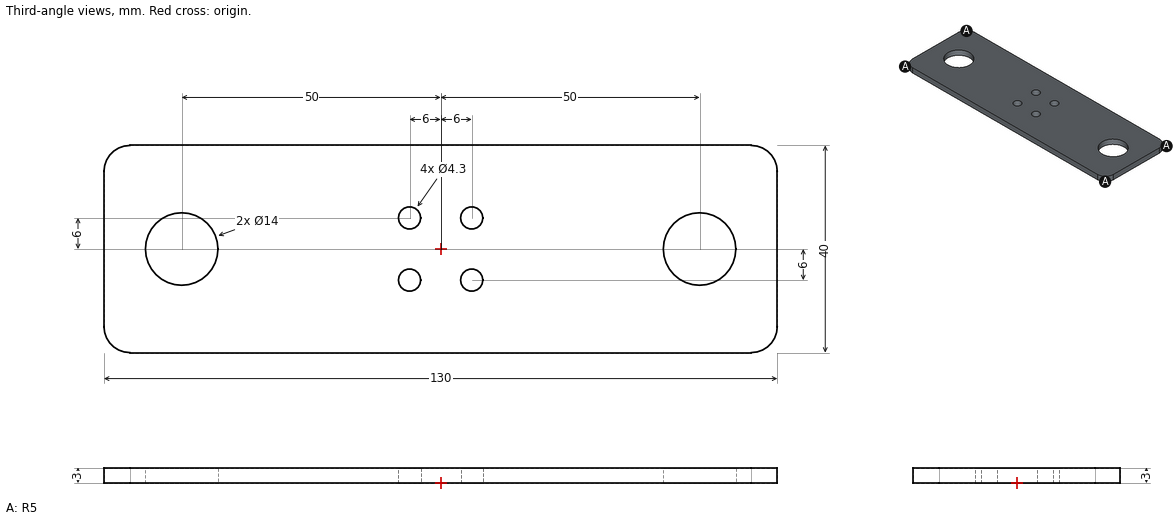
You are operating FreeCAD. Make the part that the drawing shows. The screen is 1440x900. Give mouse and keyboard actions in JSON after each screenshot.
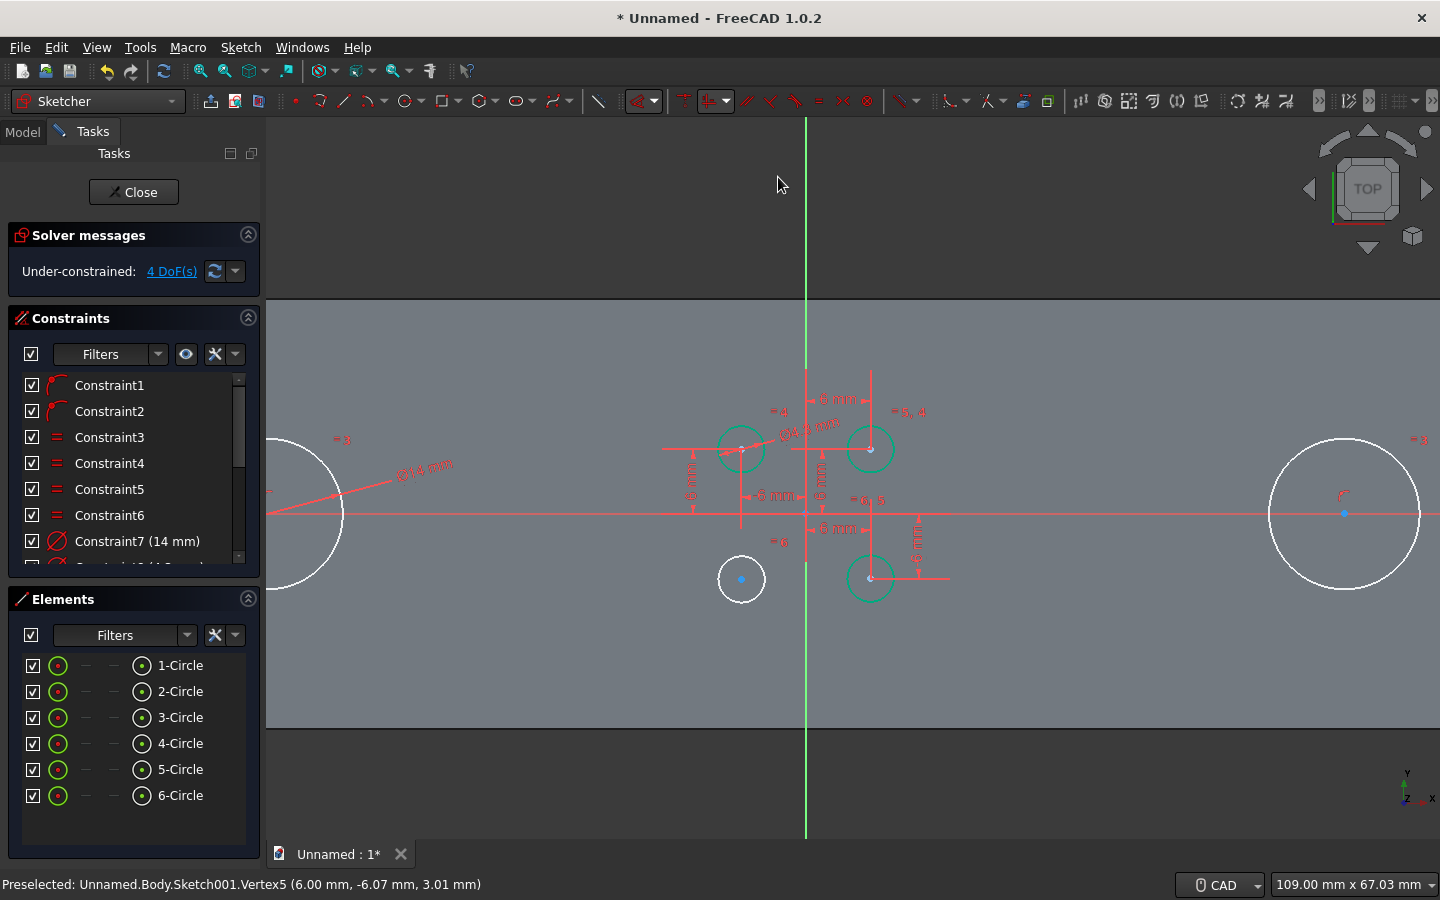
{"action": "left_click", "coordinate": [742, 579]}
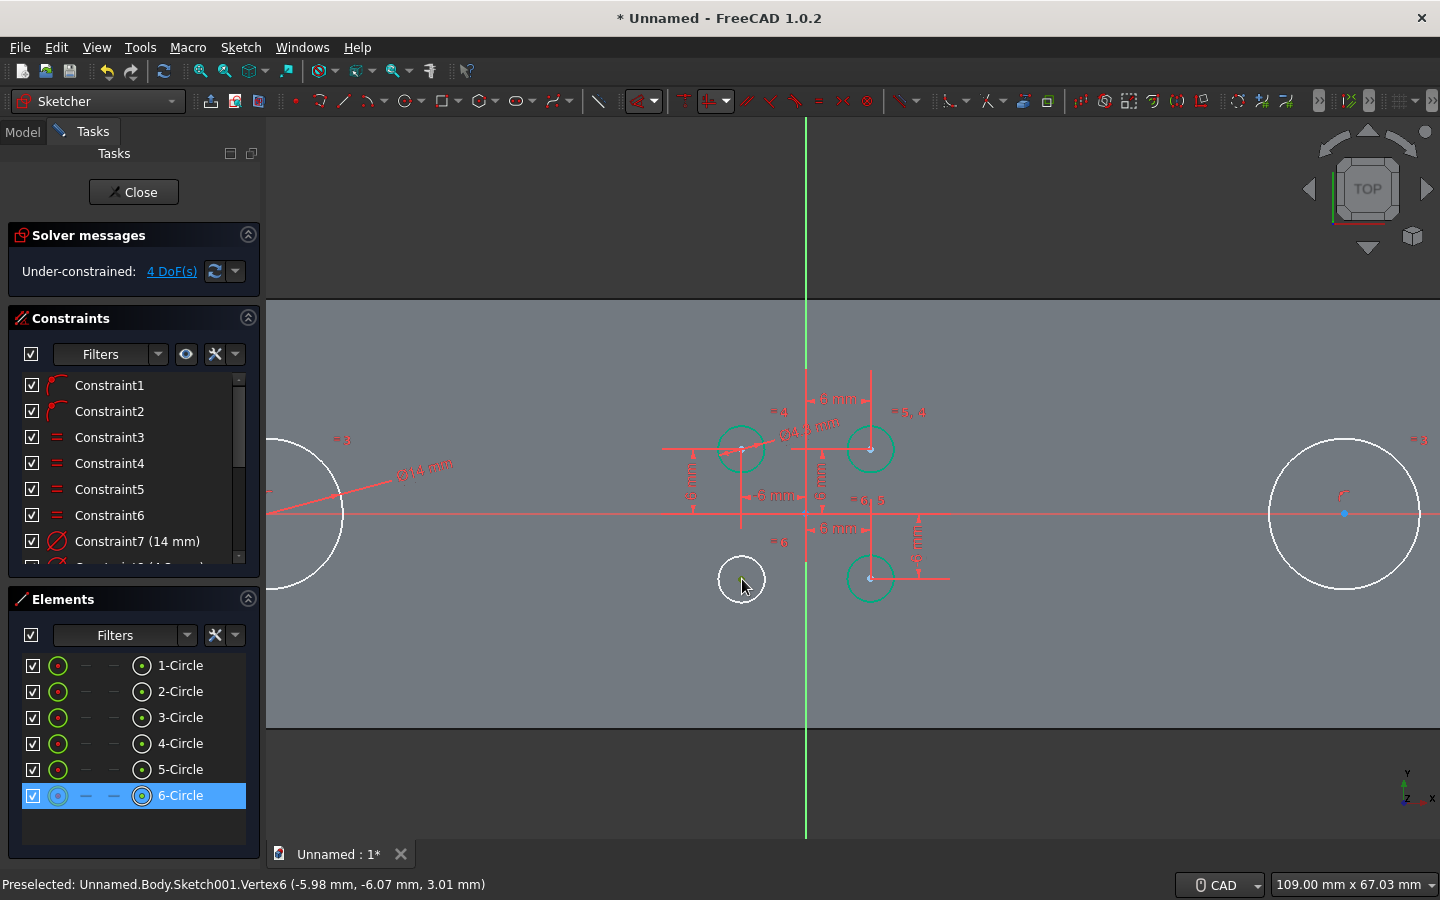
{"action": "key", "text": "l"}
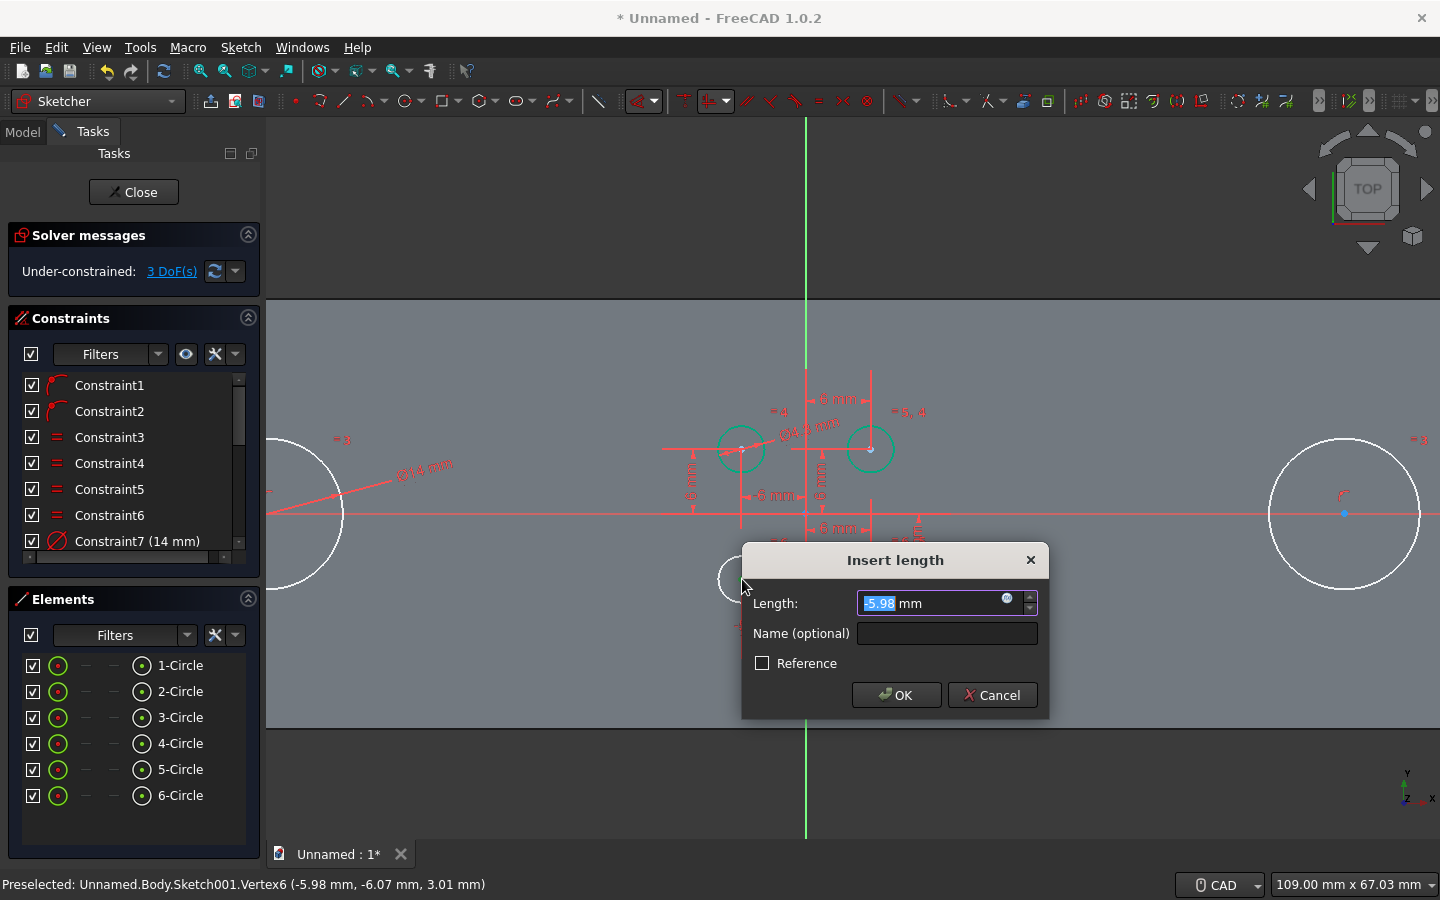
{"action": "type", "text": "-6"}
{"action": "key", "text": "Return"}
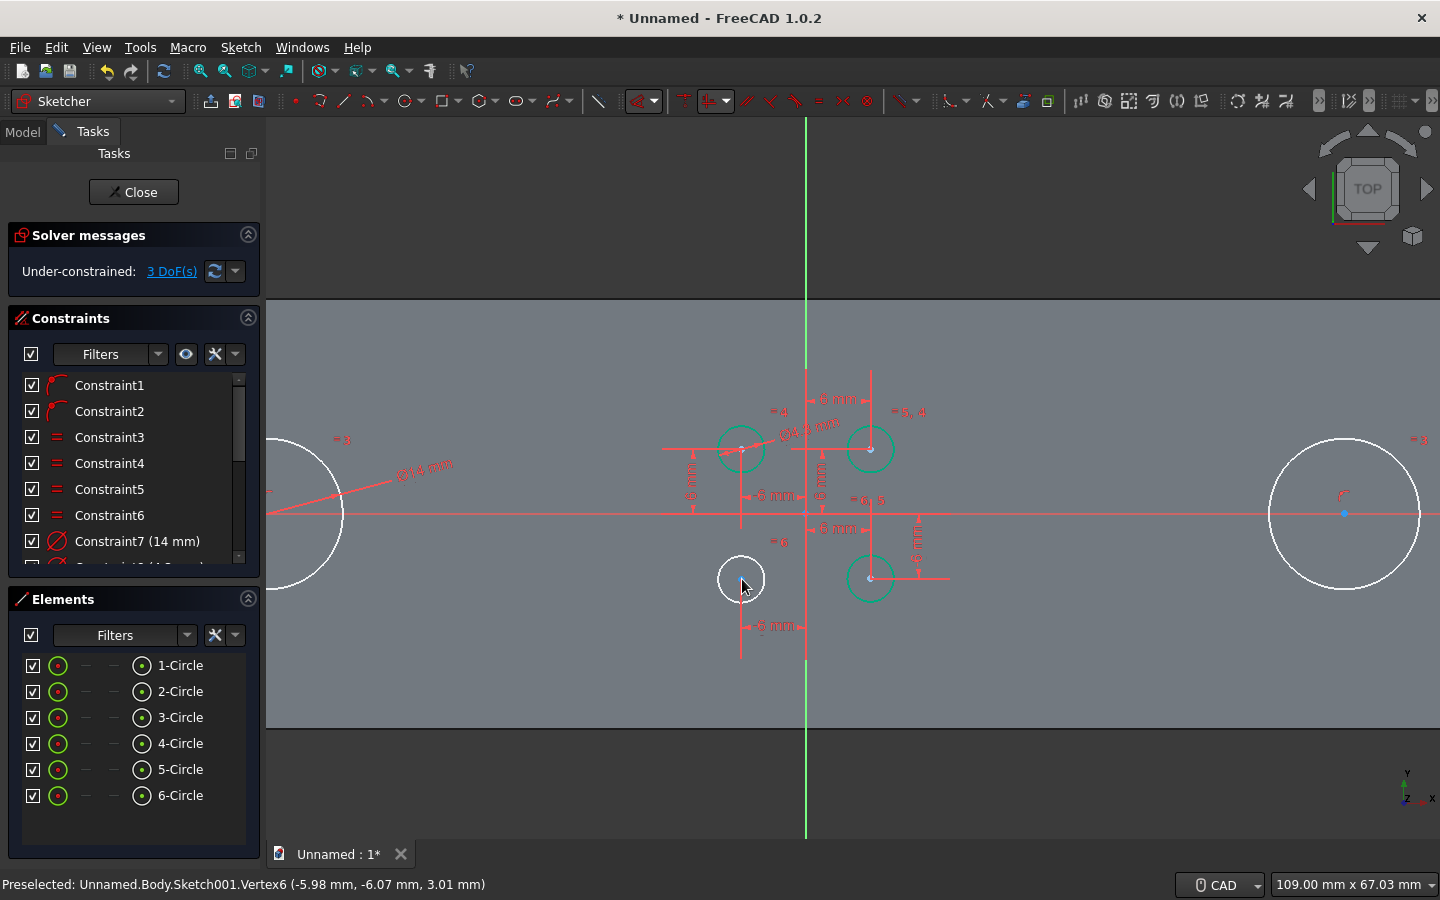
{"action": "left_click", "coordinate": [741, 579]}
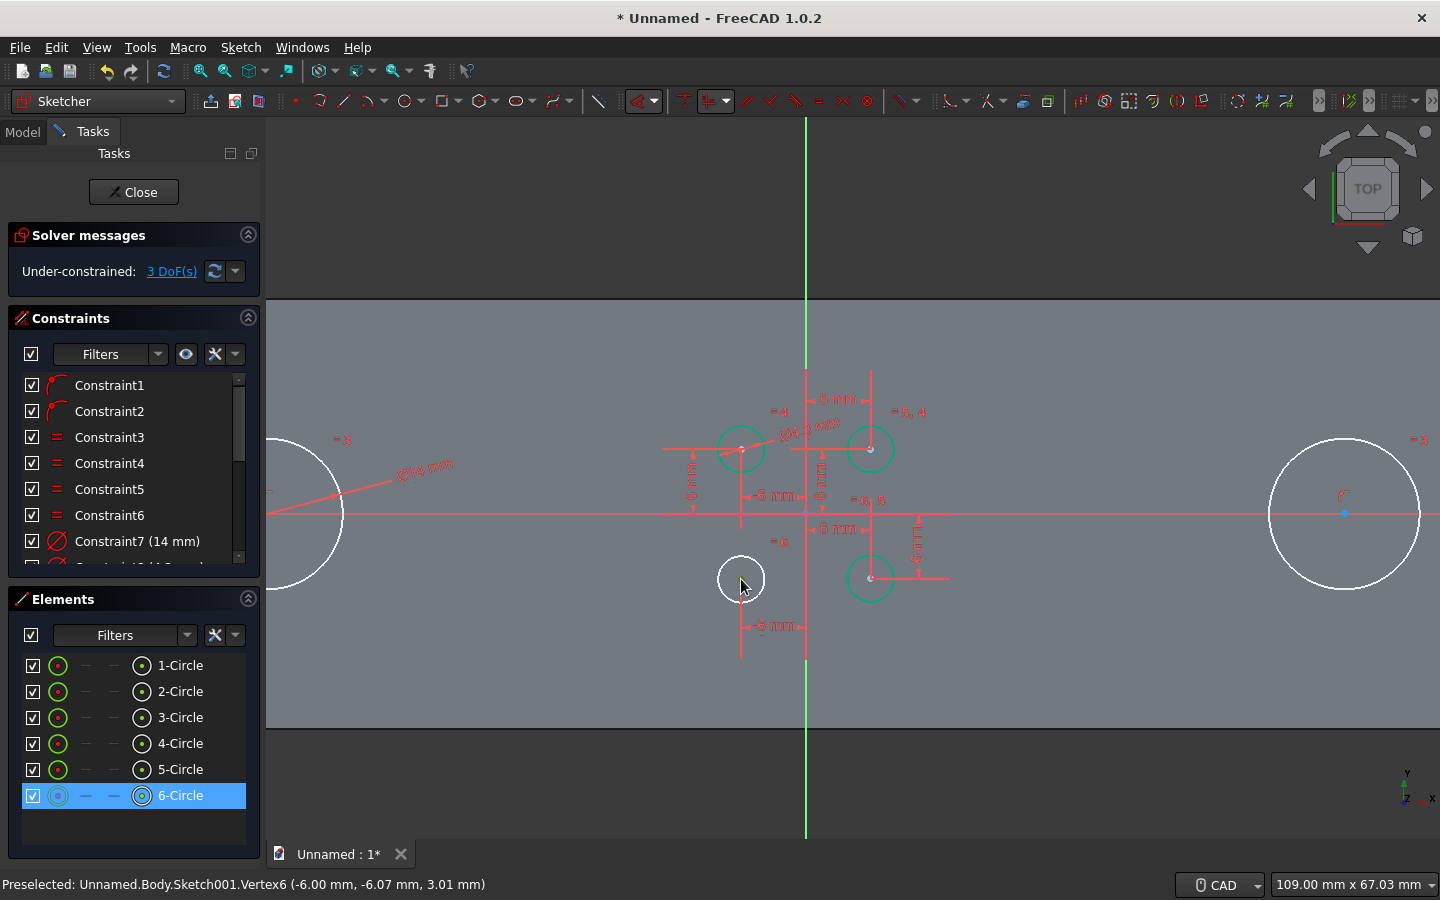
{"action": "left_click", "coordinate": [656, 102]}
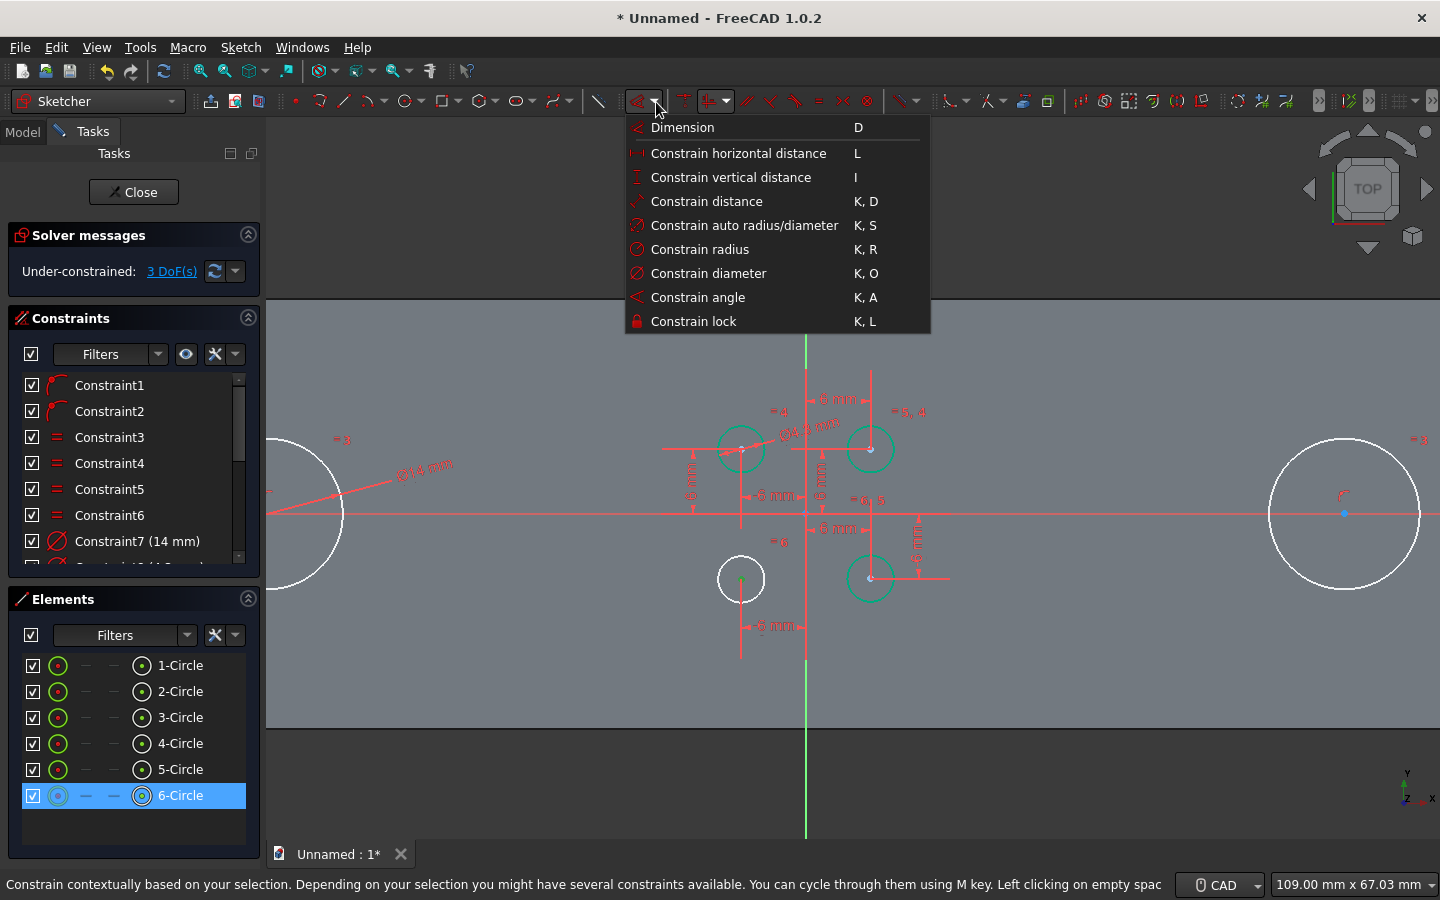
{"action": "left_click", "coordinate": [778, 177]}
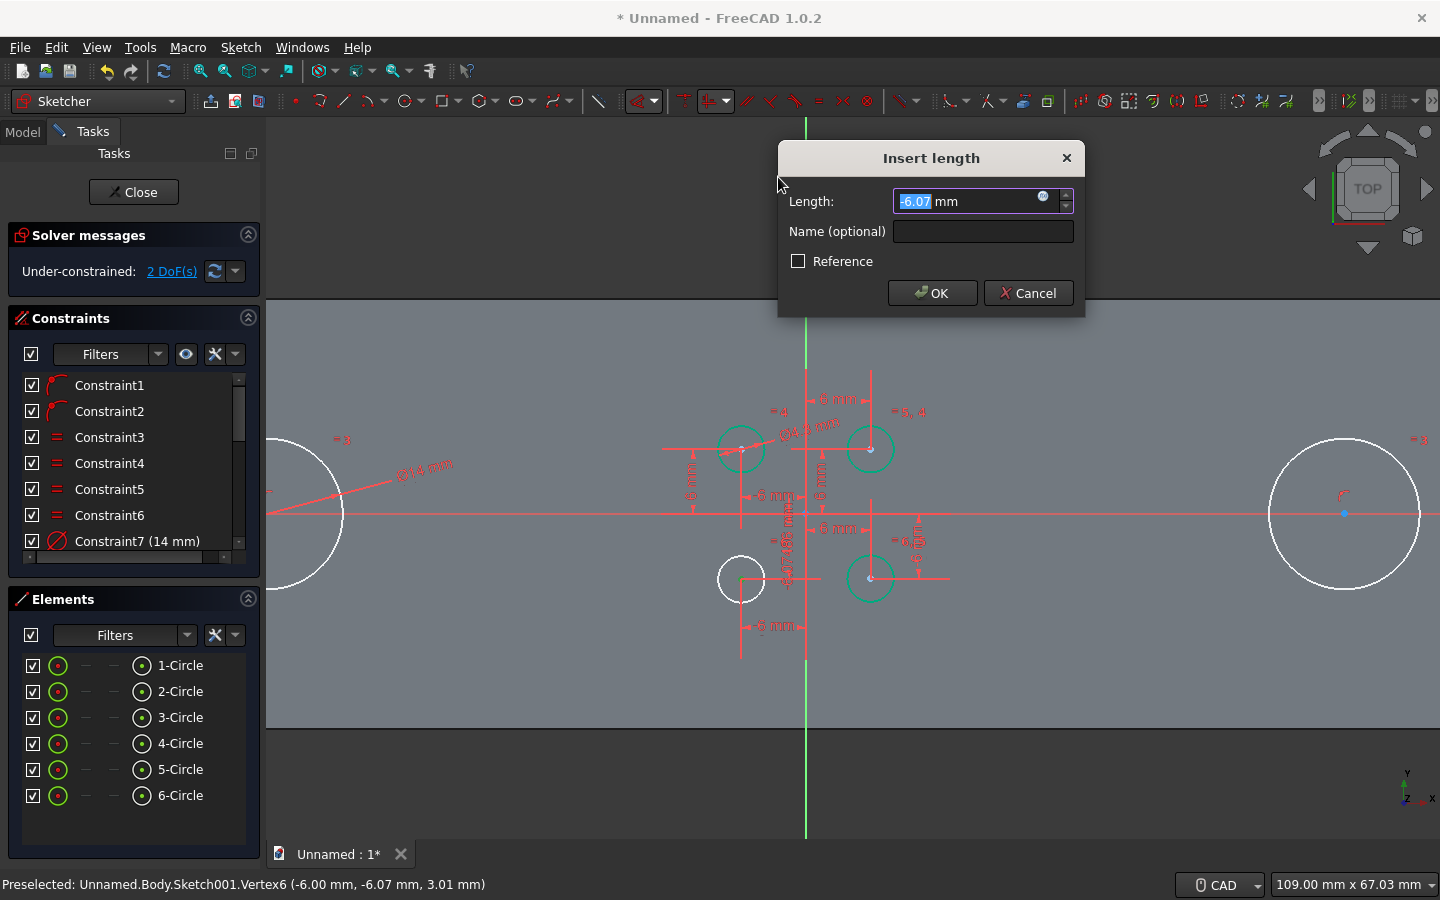
{"action": "type", "text": "-6"}
{"action": "key", "text": "Return"}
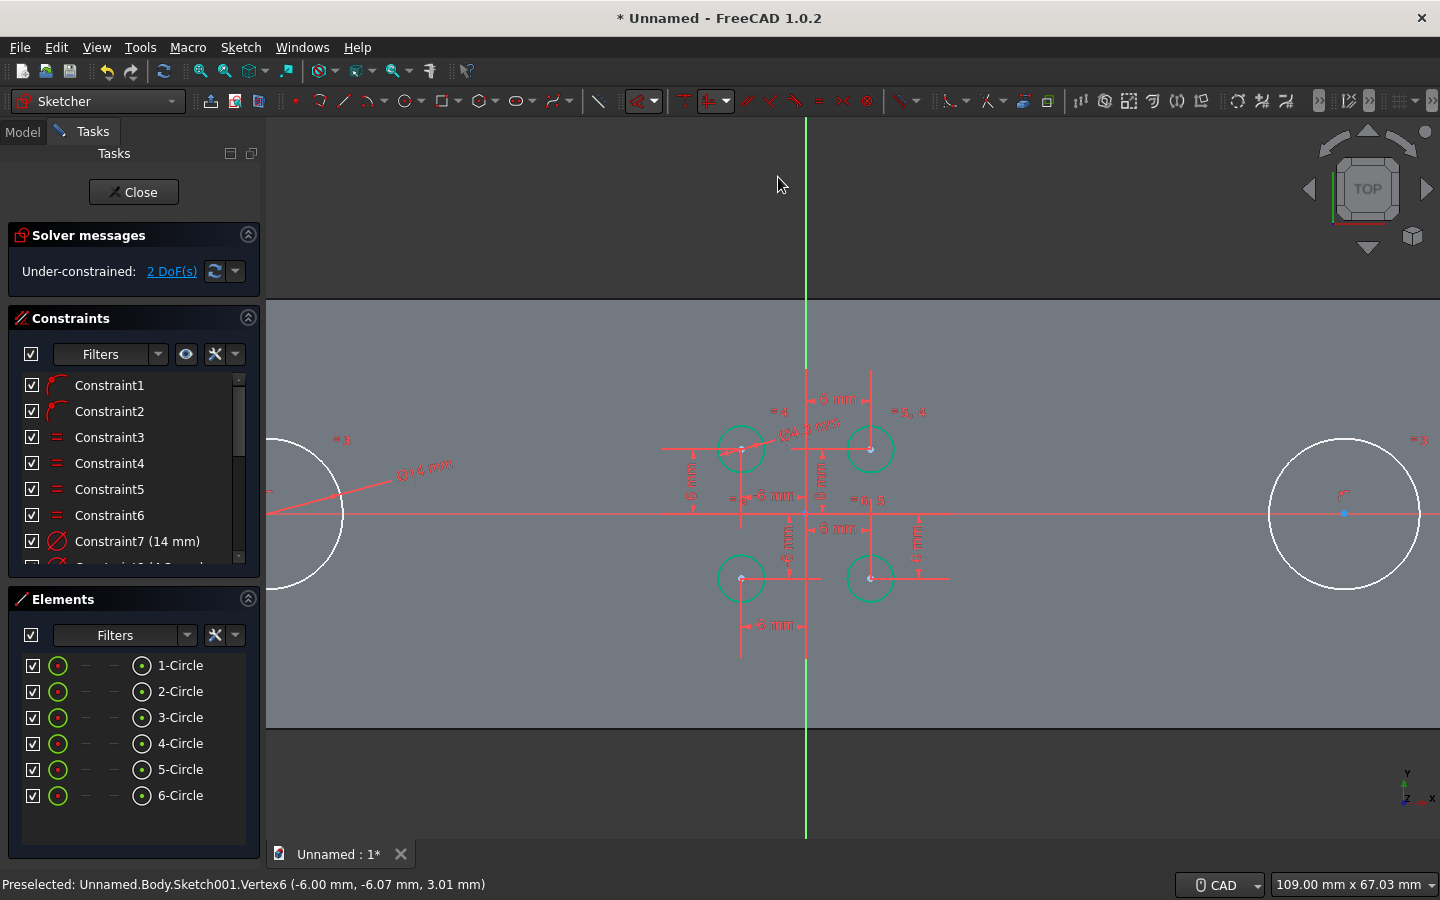
{"action": "scroll", "coordinate": [758, 434], "scroll_direction": "down", "scroll_amount": 3}